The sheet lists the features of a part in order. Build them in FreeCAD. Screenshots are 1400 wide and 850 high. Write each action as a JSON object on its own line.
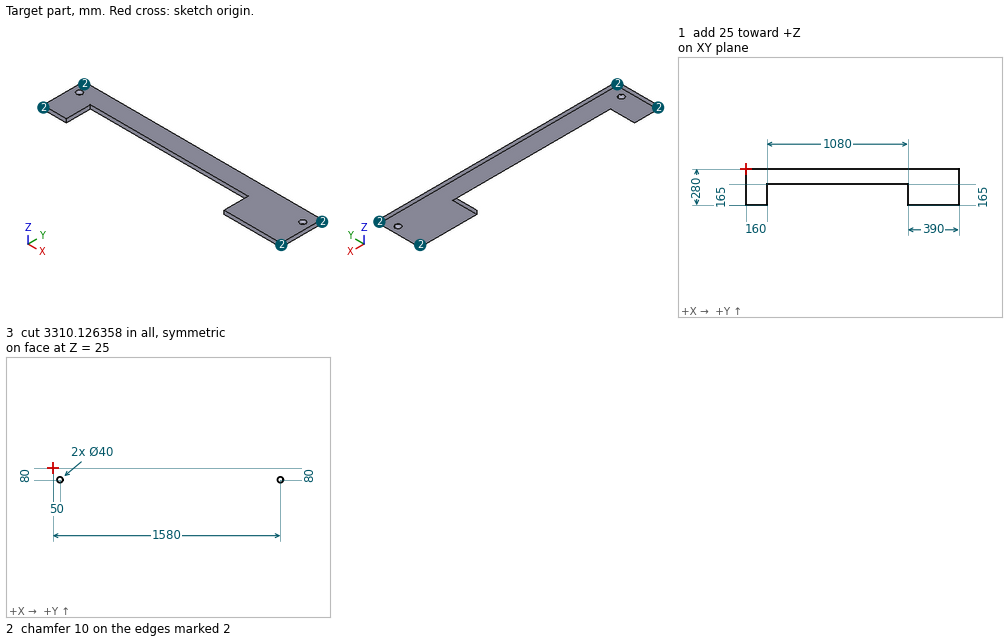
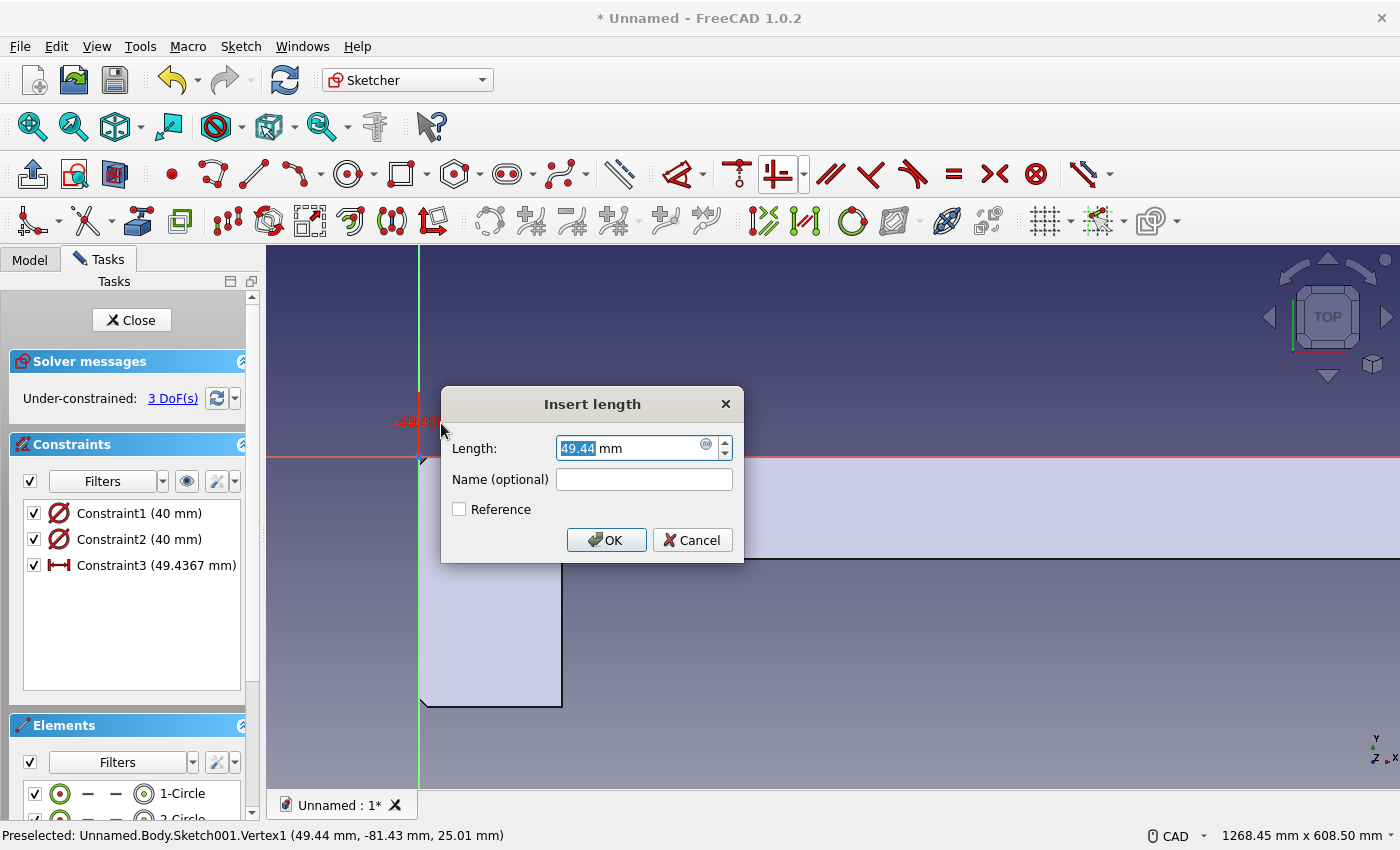
{"action": "type", "text": "50"}
{"action": "key", "text": "Return"}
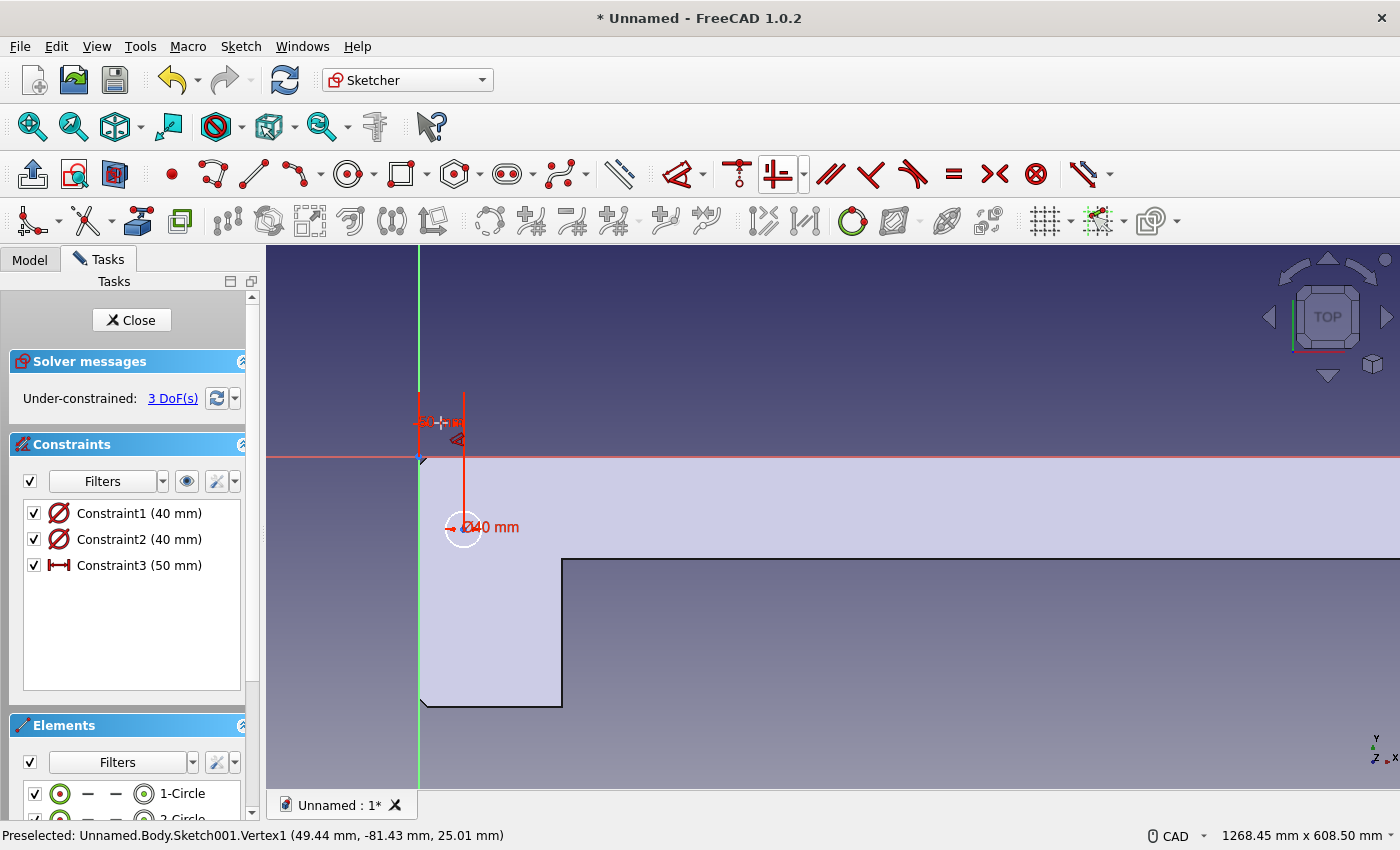
{"action": "left_click", "coordinate": [464, 529]}
{"action": "left_click", "coordinate": [385, 493]}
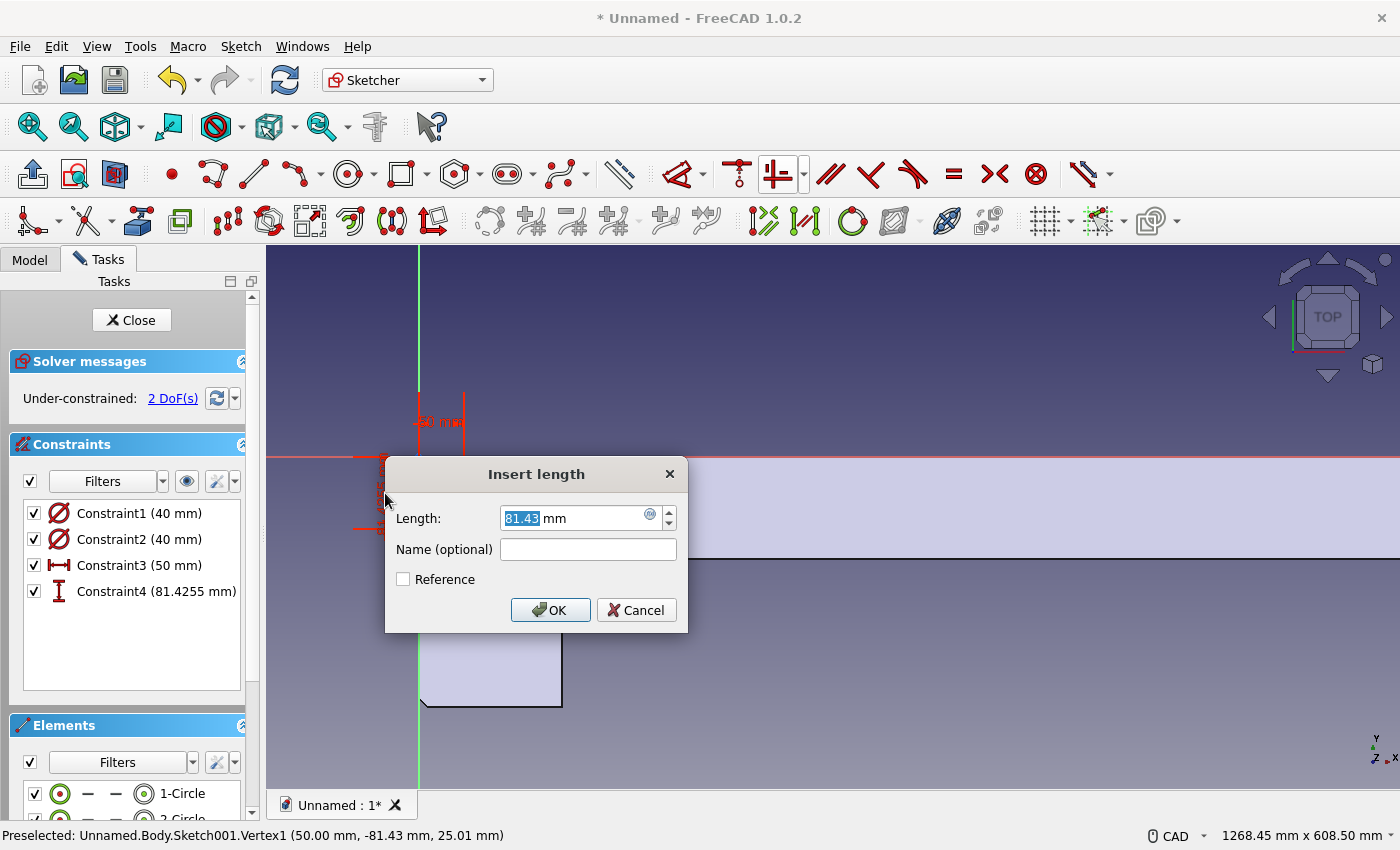
{"action": "type", "text": "80"}
{"action": "key", "text": "Return"}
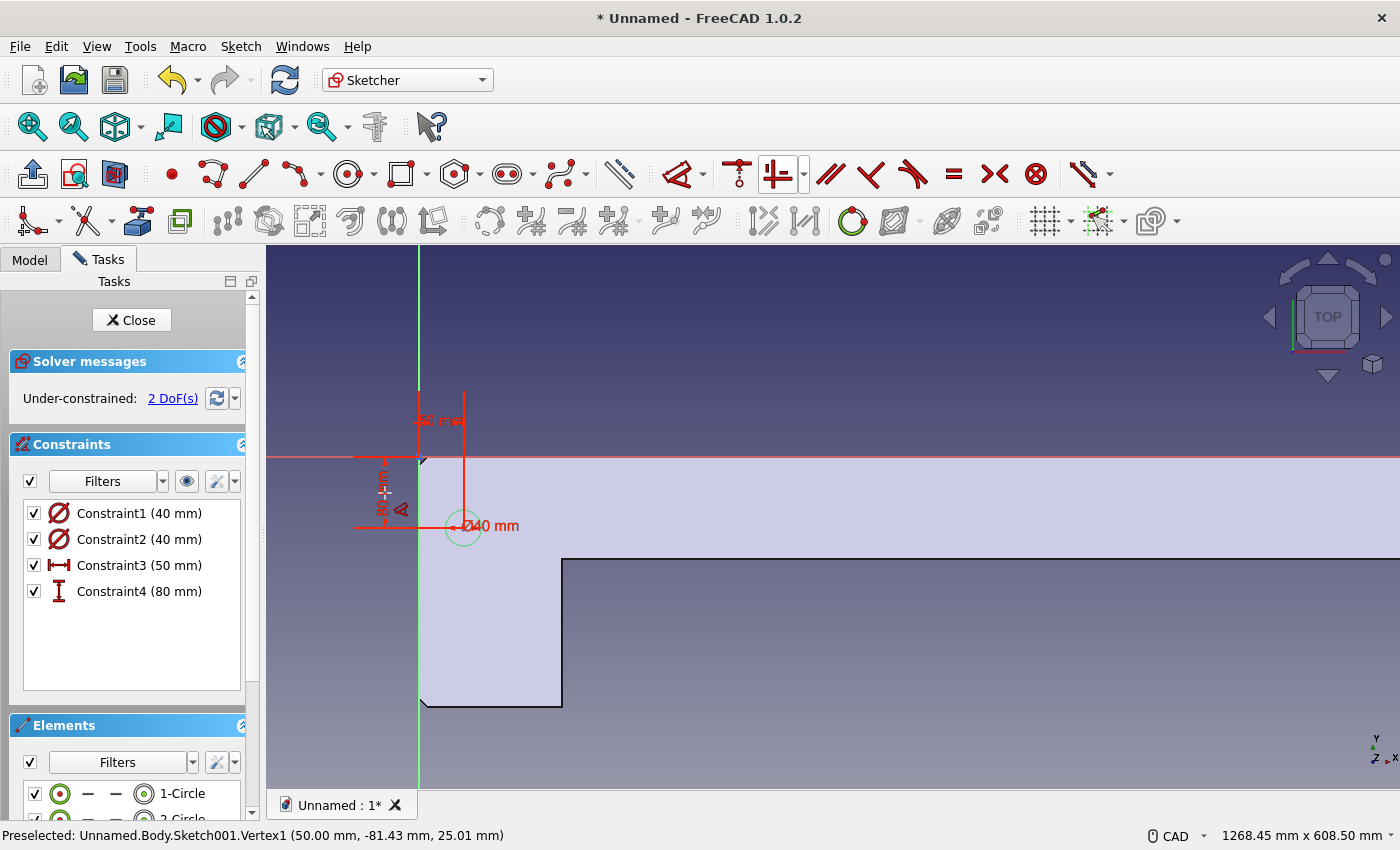
{"action": "scroll", "coordinate": [463, 530], "scroll_direction": "down", "scroll_amount": 4}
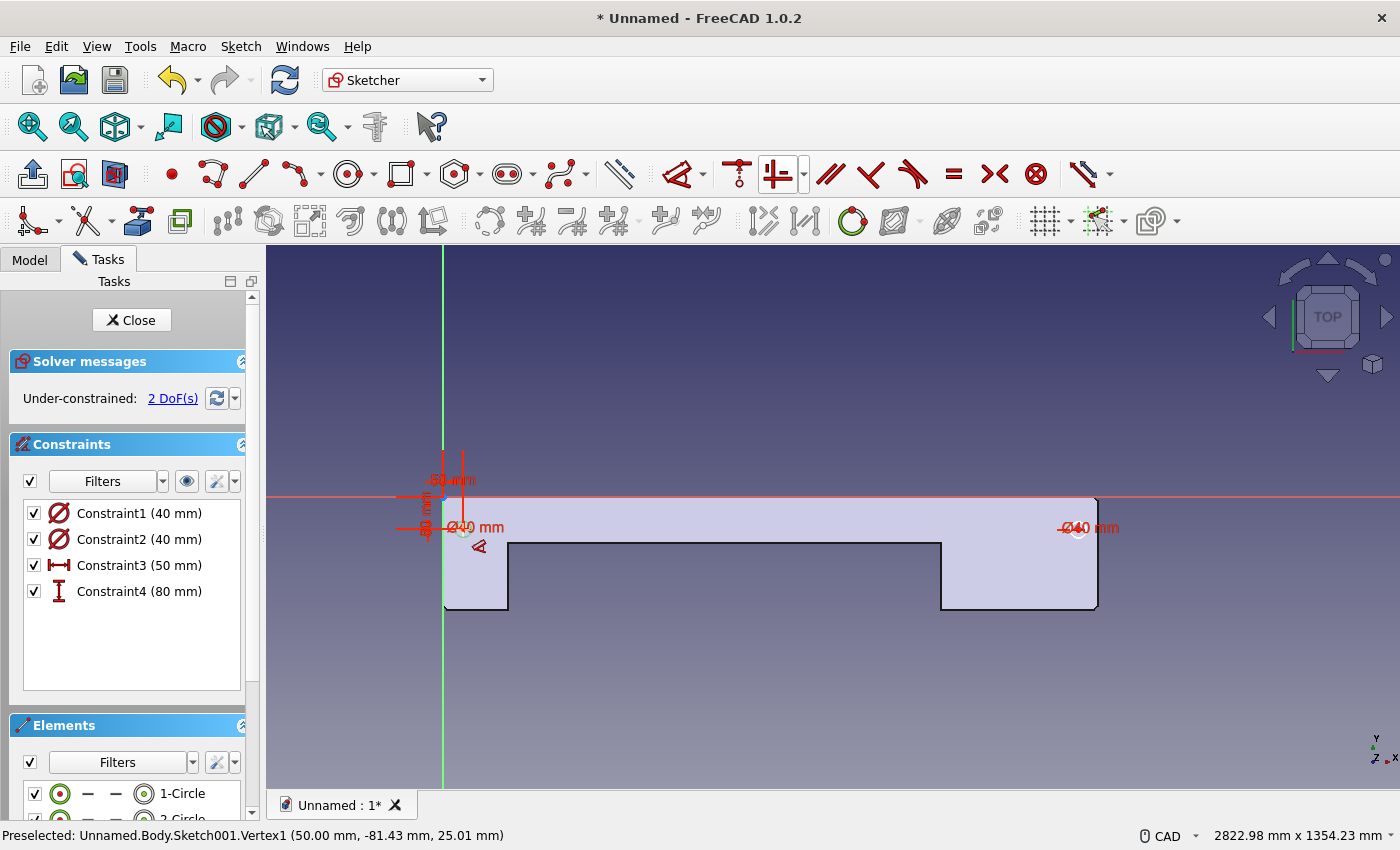
{"action": "scroll", "coordinate": [1078, 530], "scroll_direction": "up", "scroll_amount": 2}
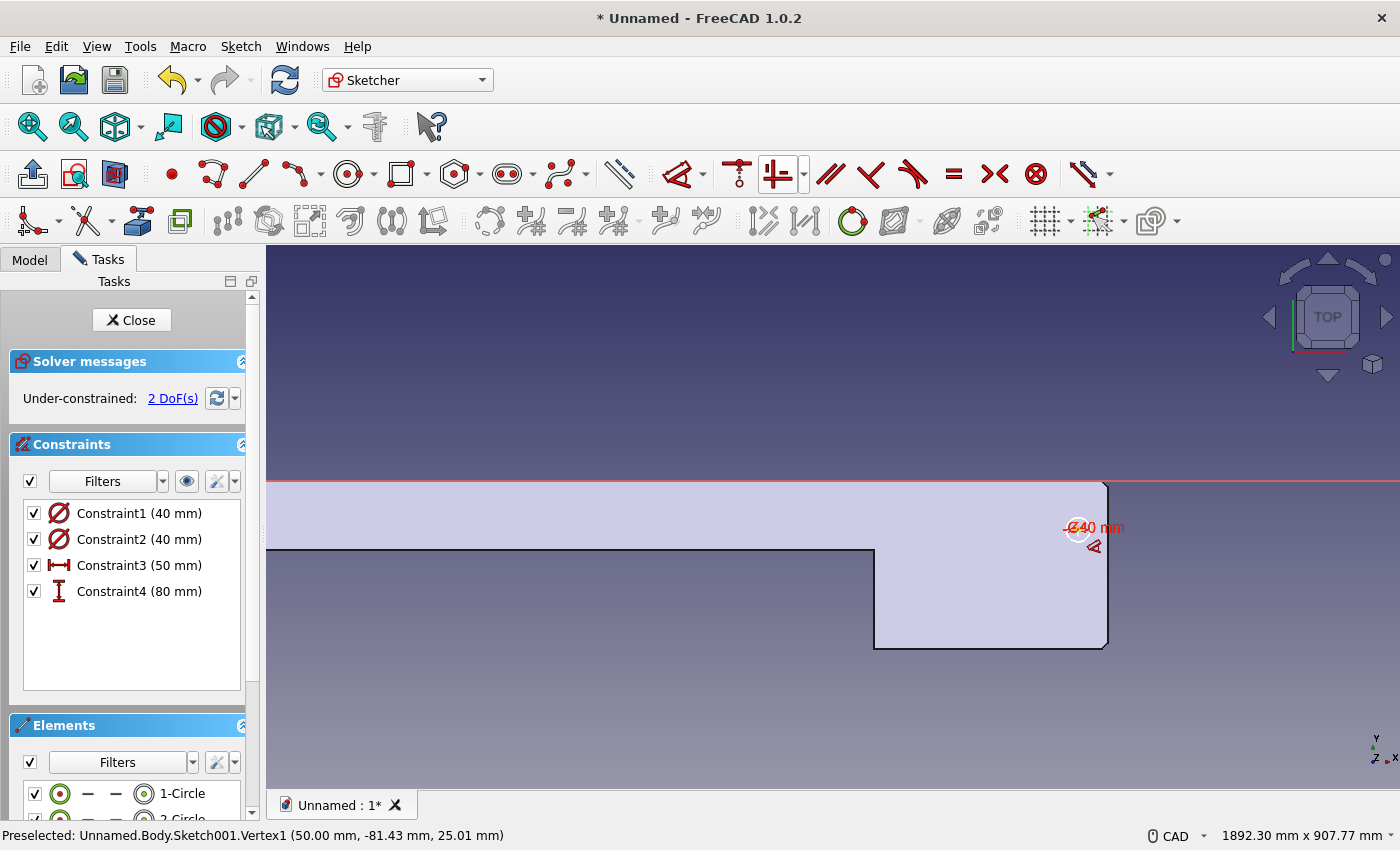
{"action": "left_click", "coordinate": [1078, 530]}
{"action": "left_click", "coordinate": [1112, 505]}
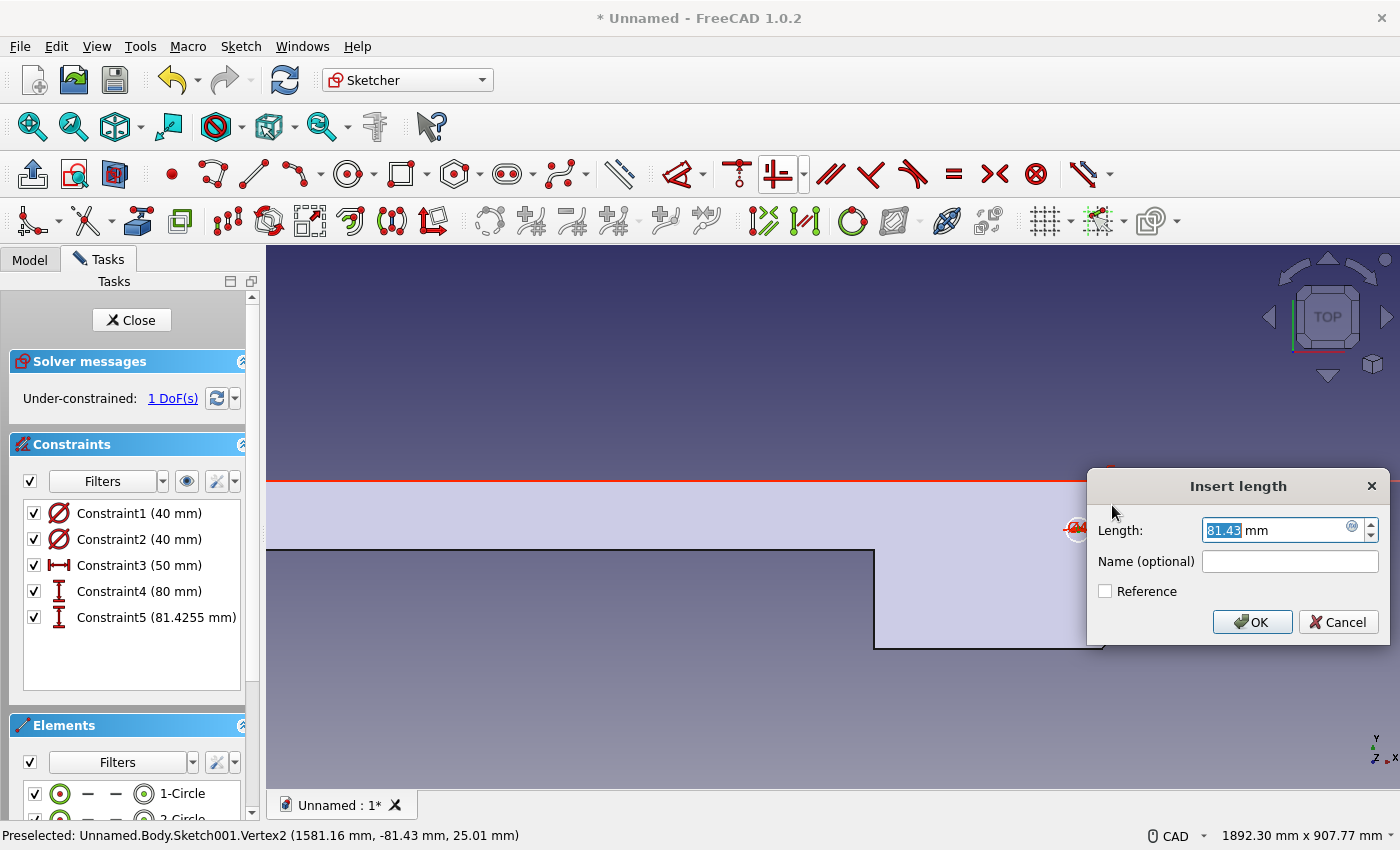
{"action": "type", "text": "80"}
{"action": "key", "text": "Return"}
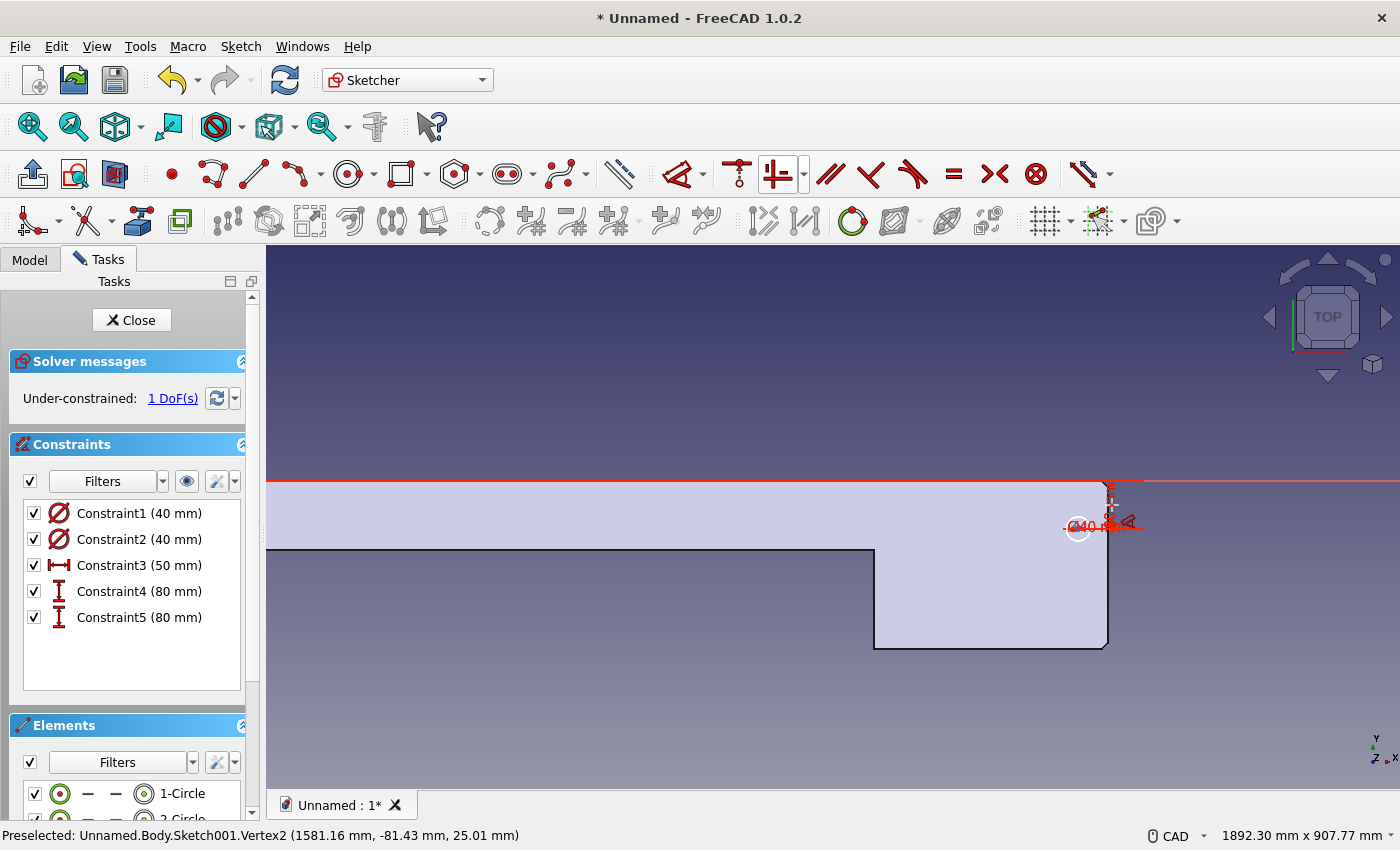
{"action": "left_click", "coordinate": [1078, 529]}
{"action": "left_click", "coordinate": [686, 447]}